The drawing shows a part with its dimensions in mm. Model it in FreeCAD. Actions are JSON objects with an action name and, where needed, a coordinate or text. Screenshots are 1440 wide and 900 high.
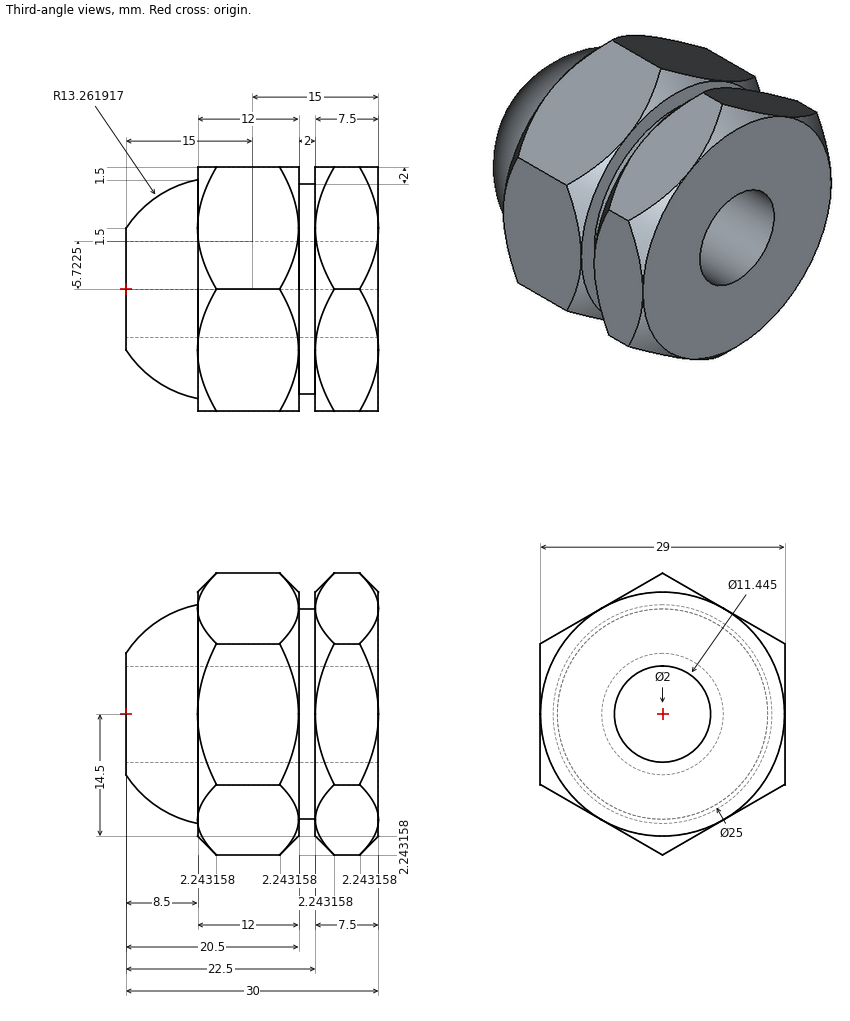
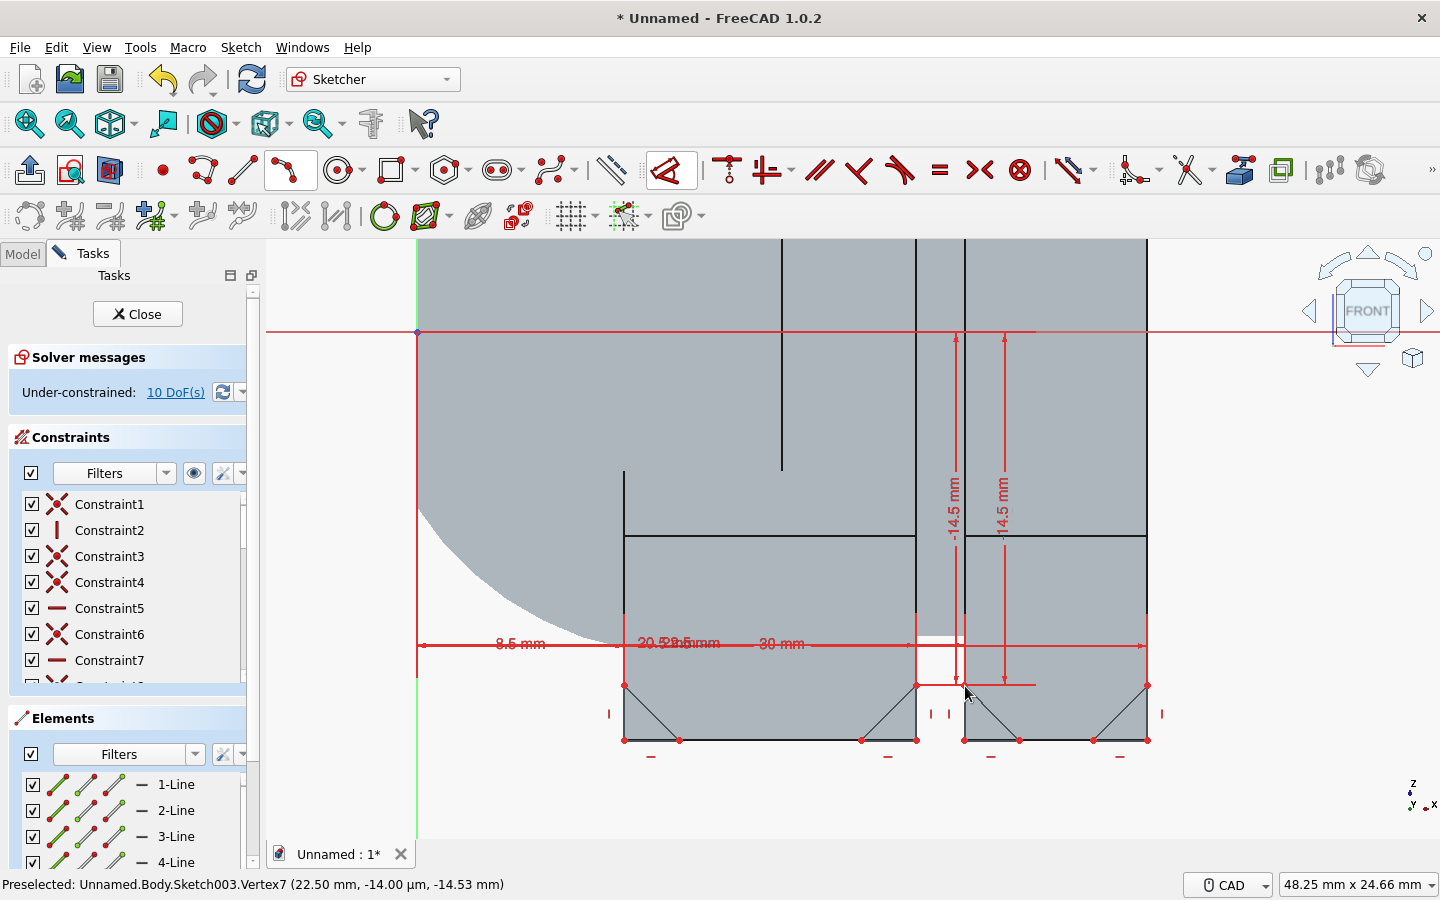
{"action": "left_click", "coordinate": [624, 686]}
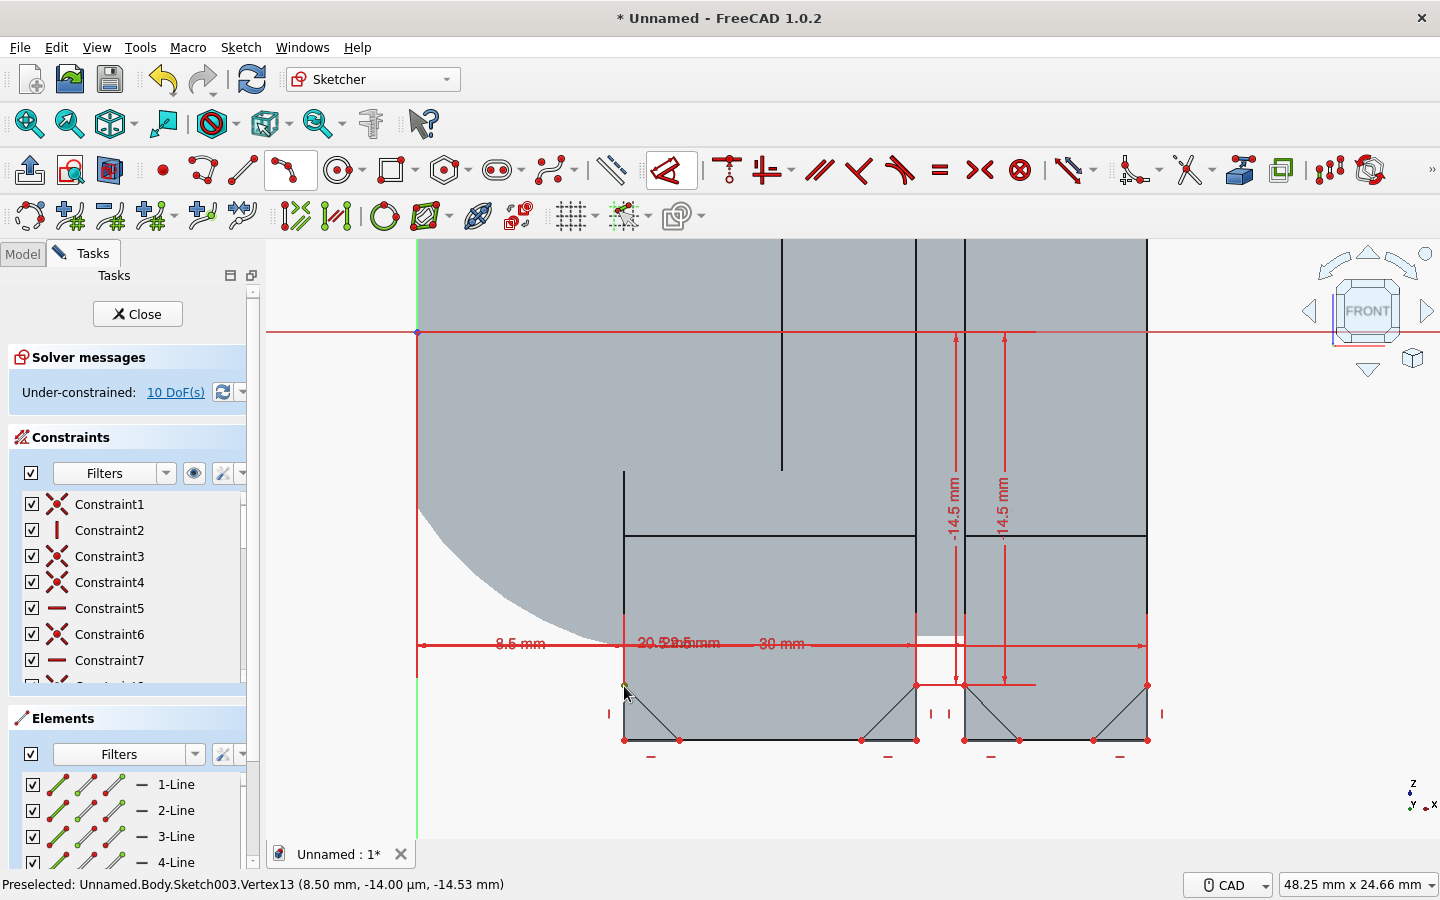
{"action": "left_click", "coordinate": [692, 170]}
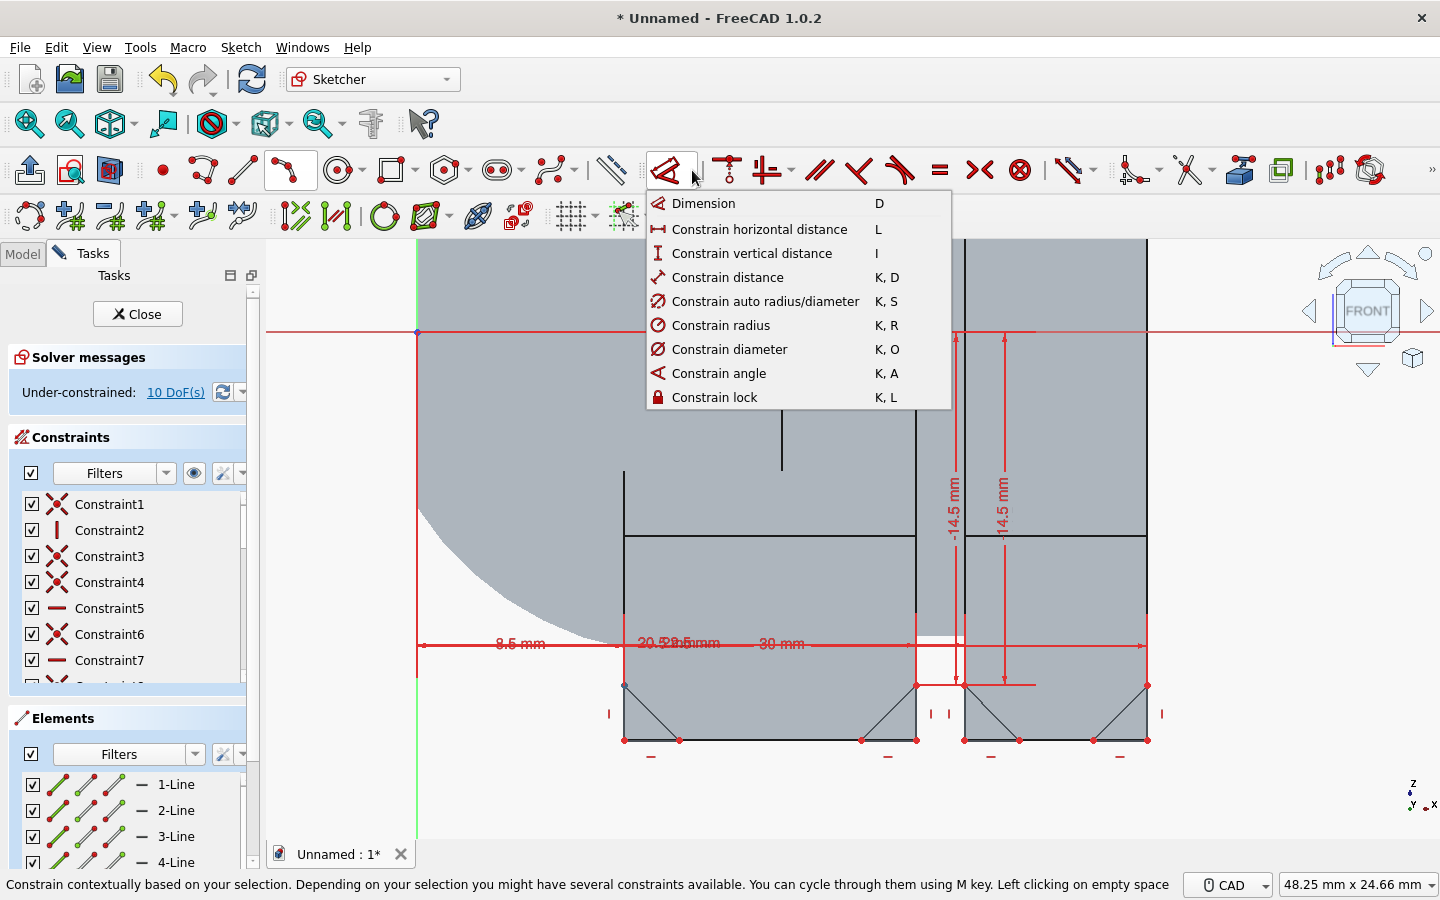
{"action": "left_click", "coordinate": [799, 253]}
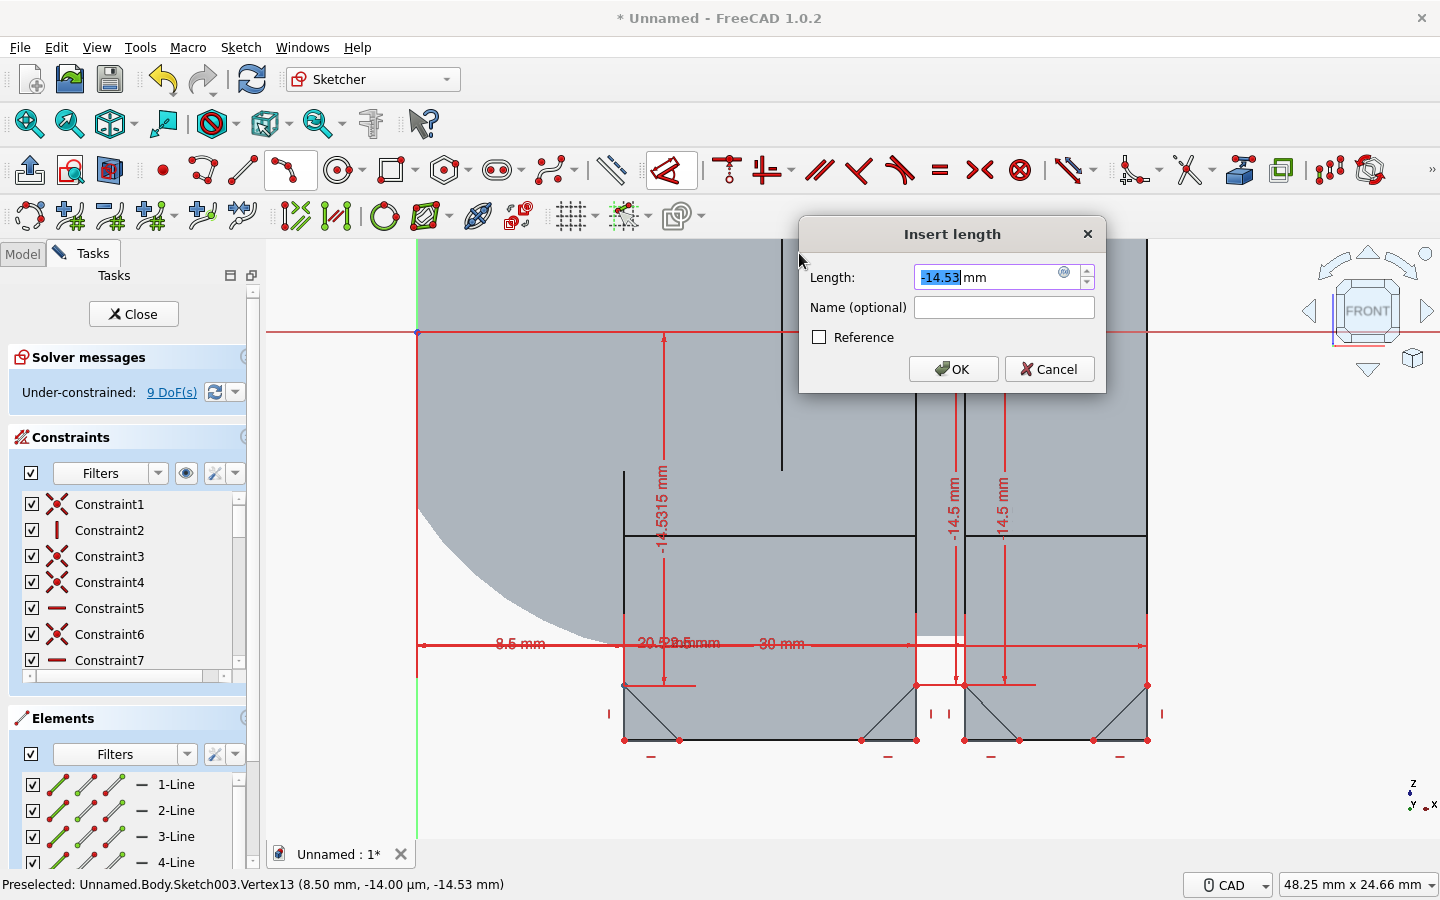
{"action": "type", "text": "-14.5"}
{"action": "key", "text": "Return"}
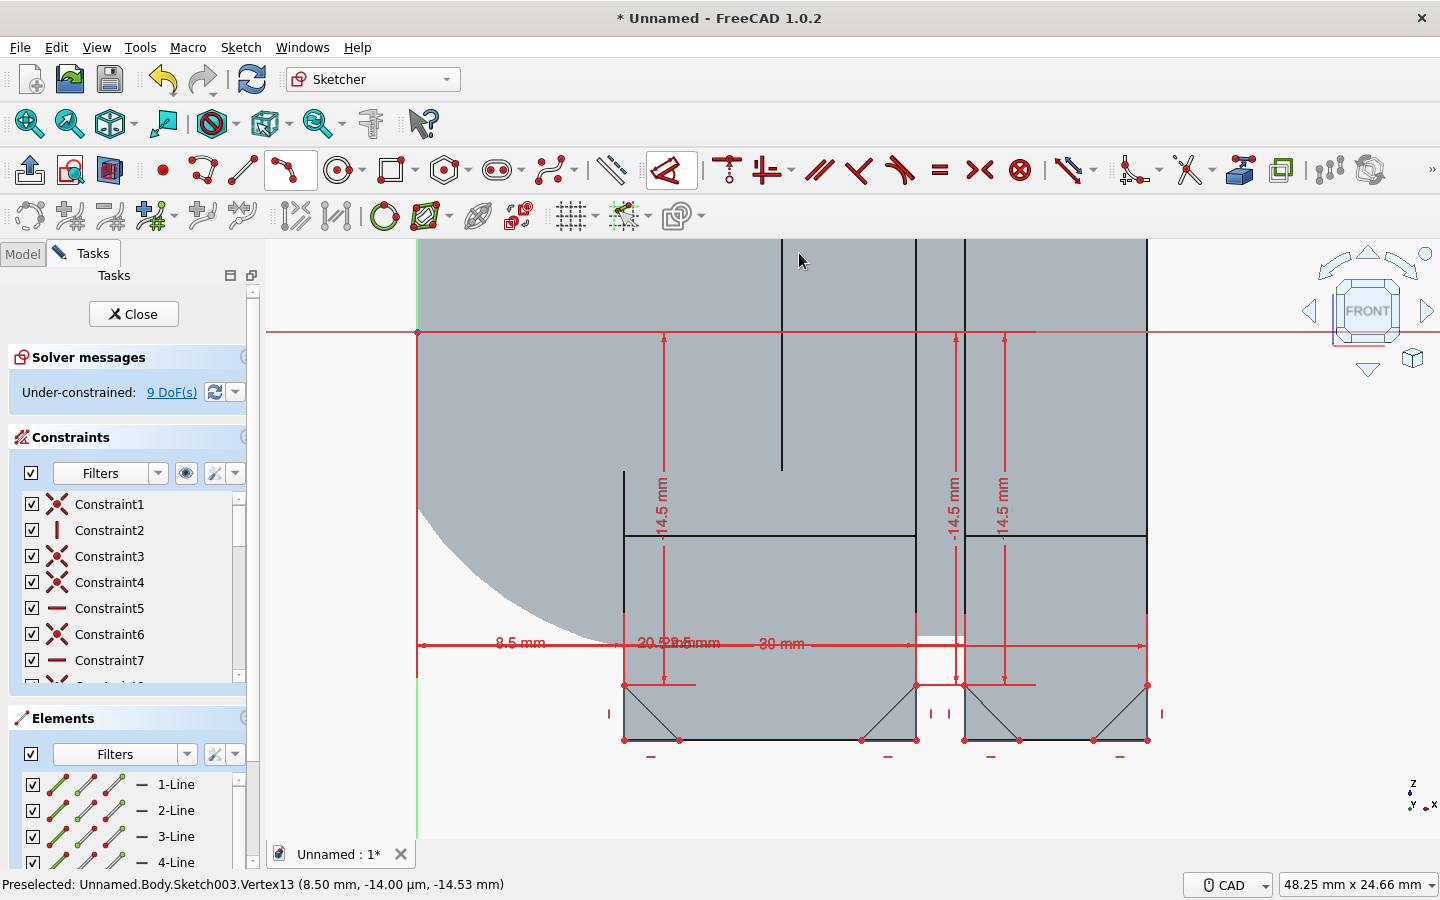
{"action": "left_click", "coordinate": [1147, 686]}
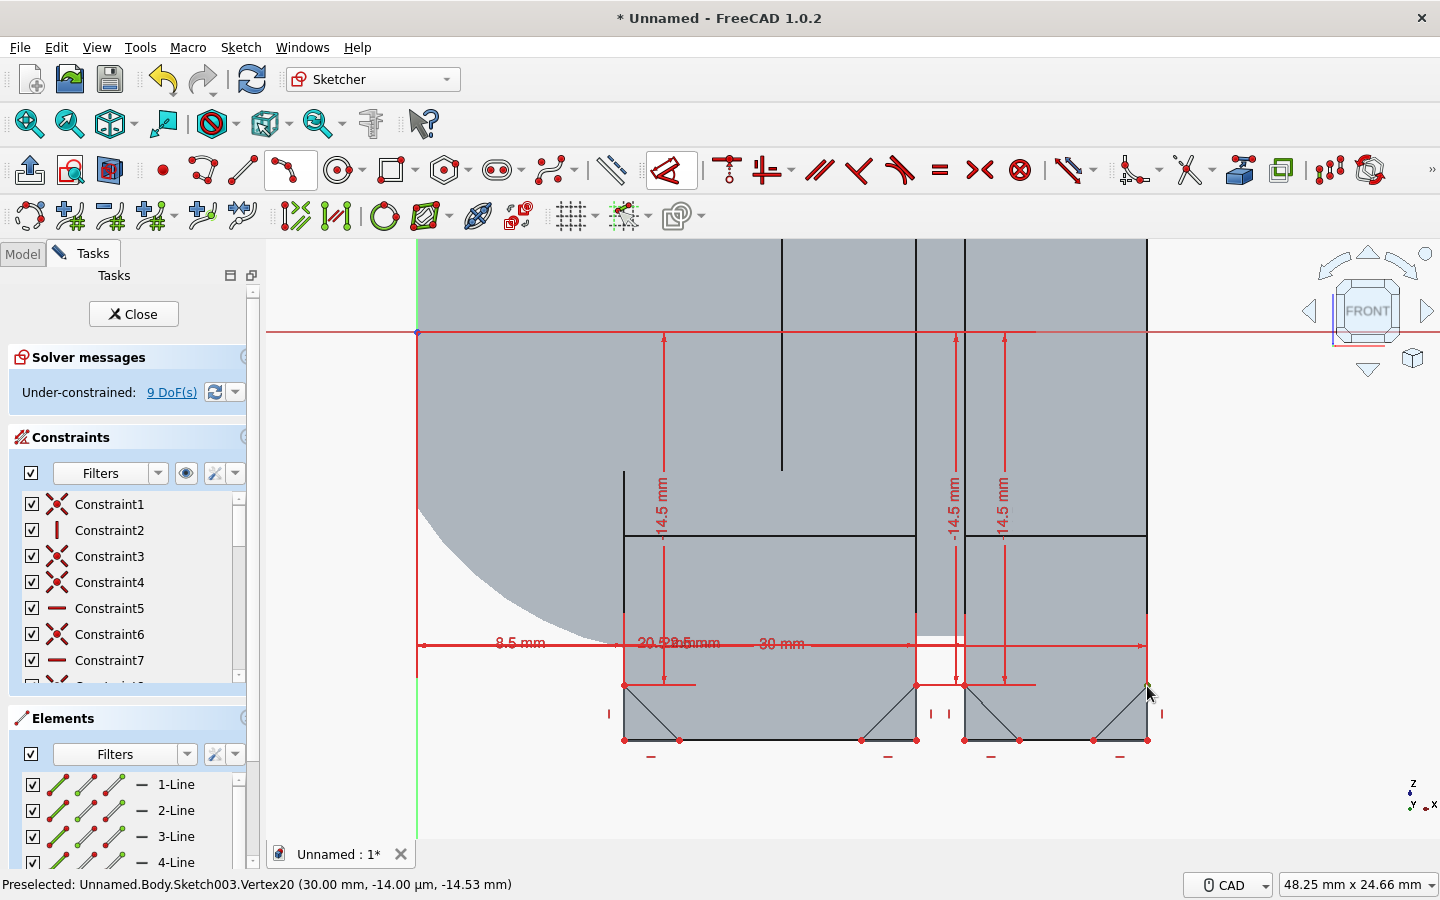
{"action": "key", "text": "i"}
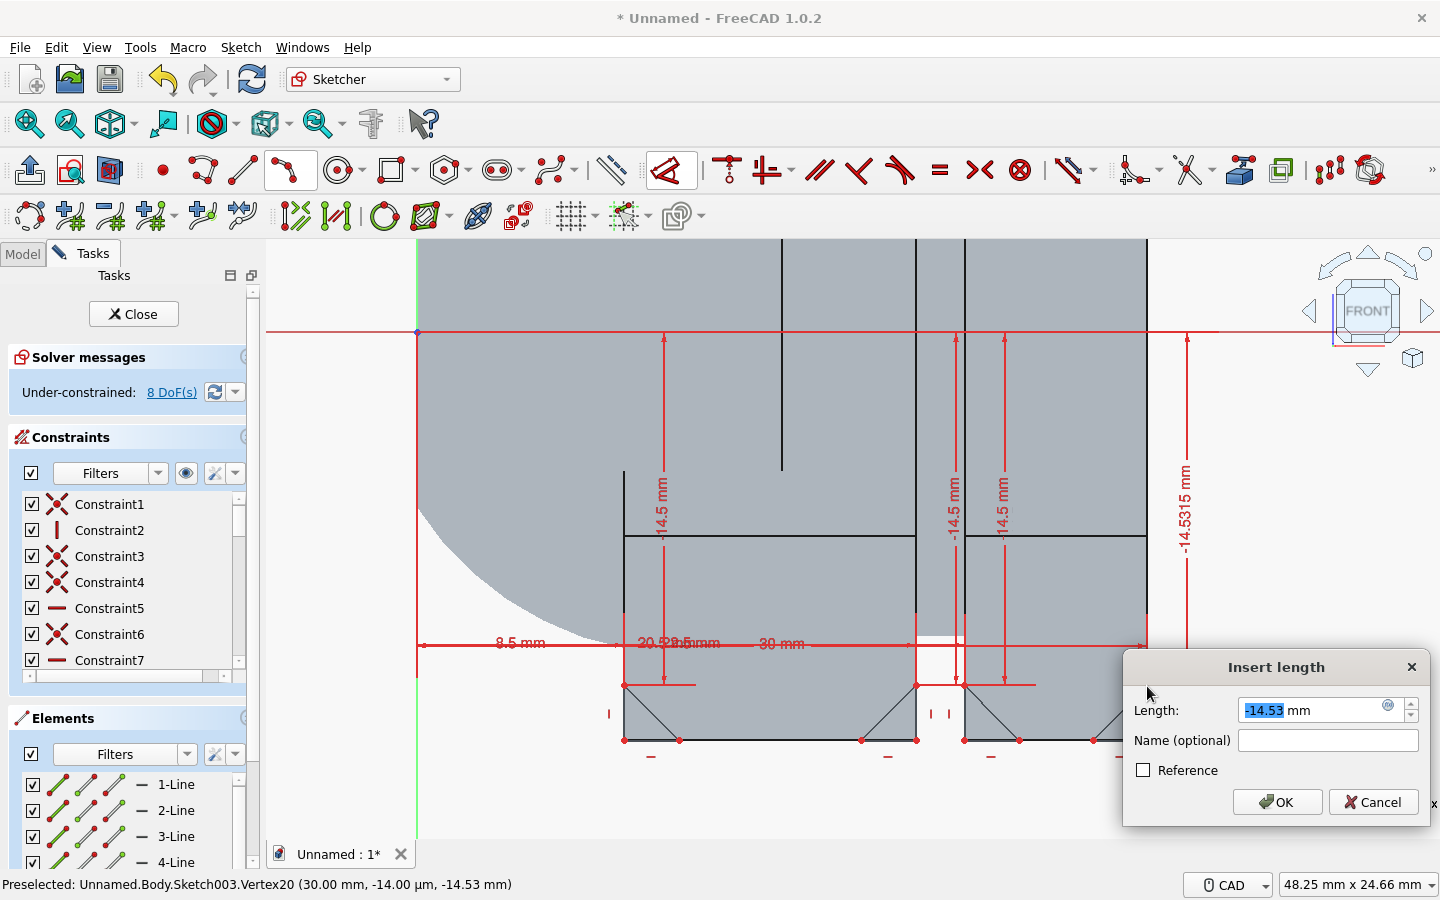
{"action": "type", "text": "-14.5"}
{"action": "key", "text": "Return"}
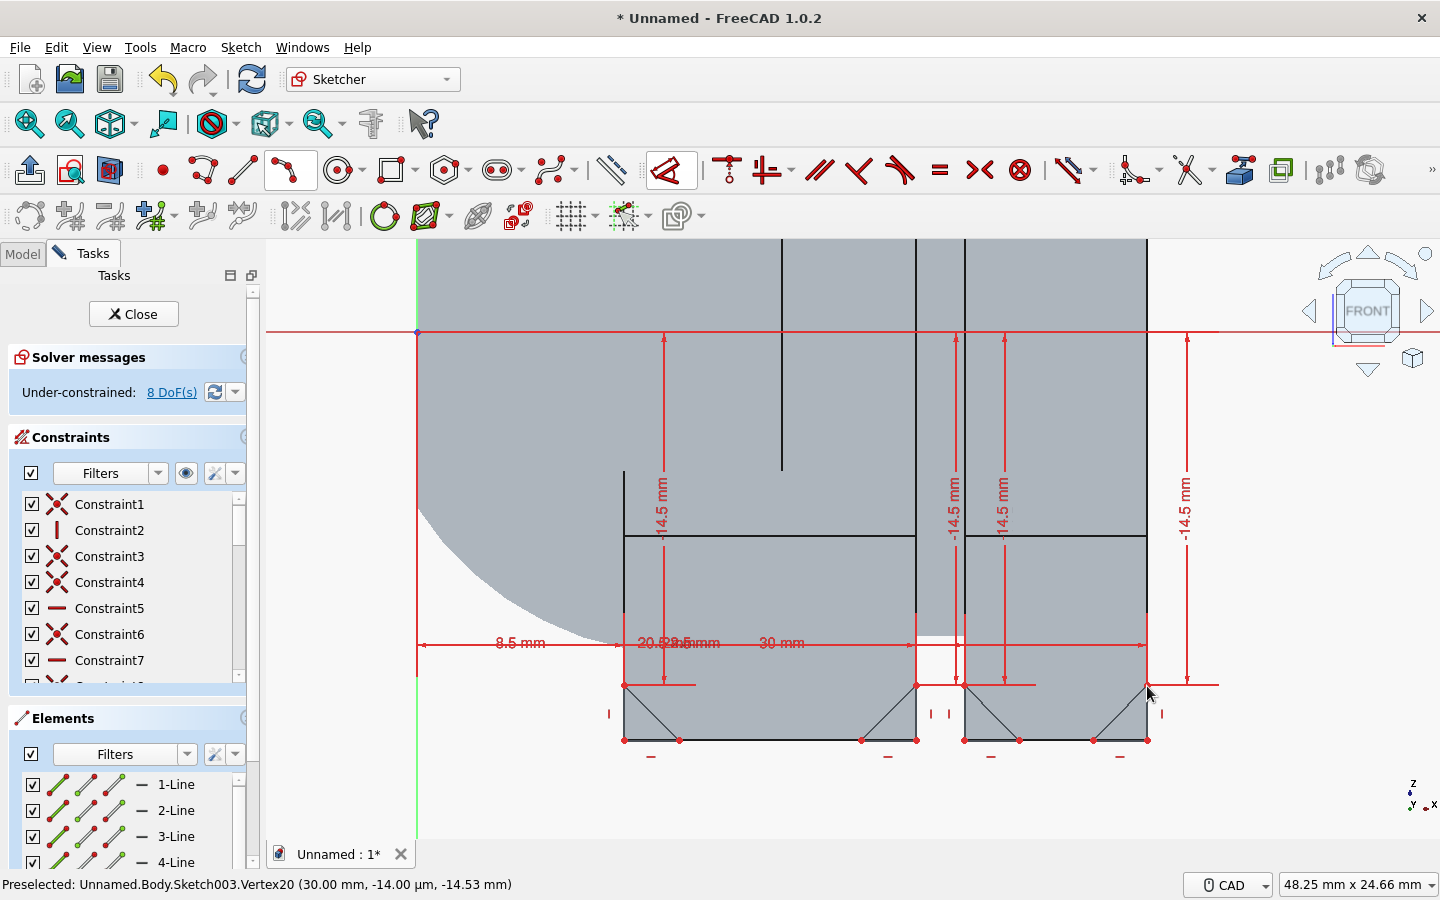
{"action": "left_click", "coordinate": [916, 702]}